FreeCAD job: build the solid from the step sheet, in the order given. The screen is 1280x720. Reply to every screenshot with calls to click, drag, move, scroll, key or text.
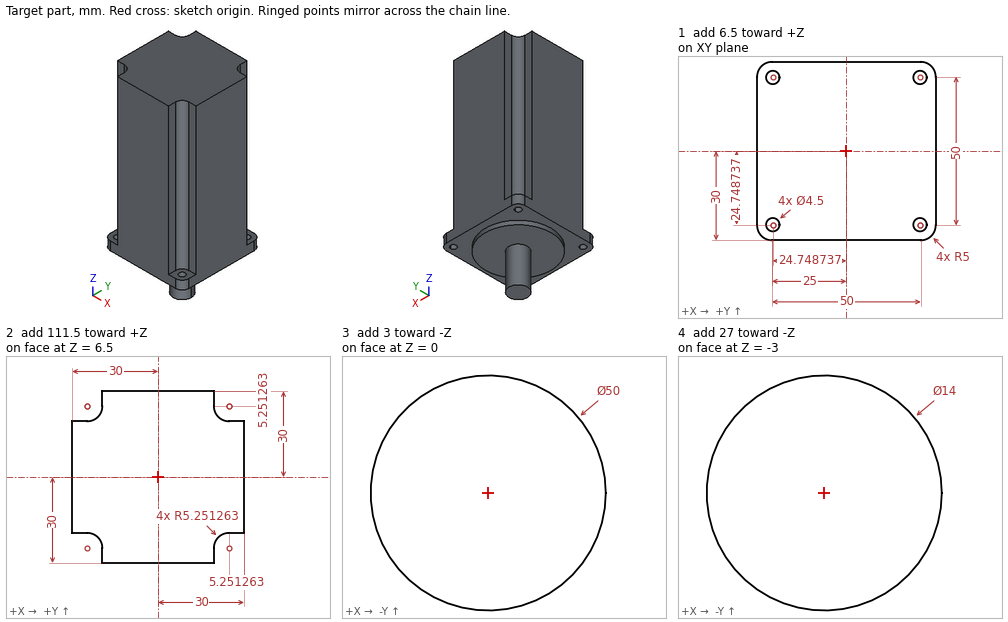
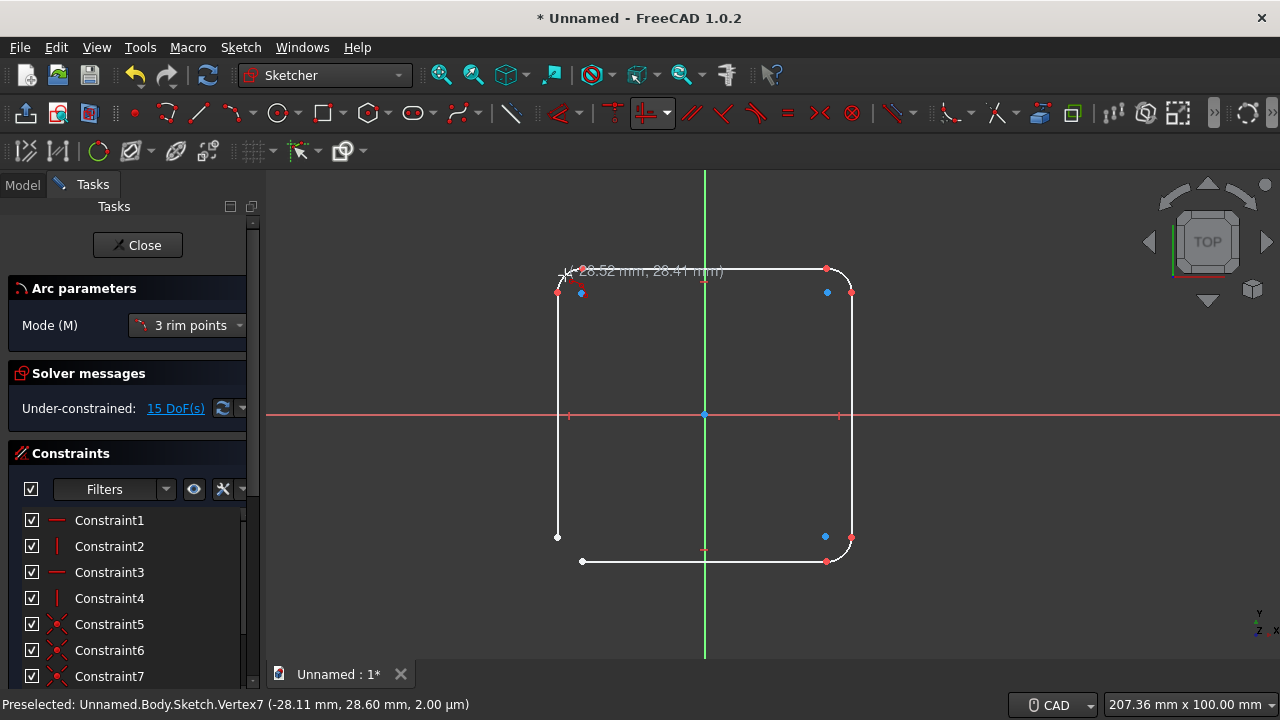
click(558, 538)
click(583, 562)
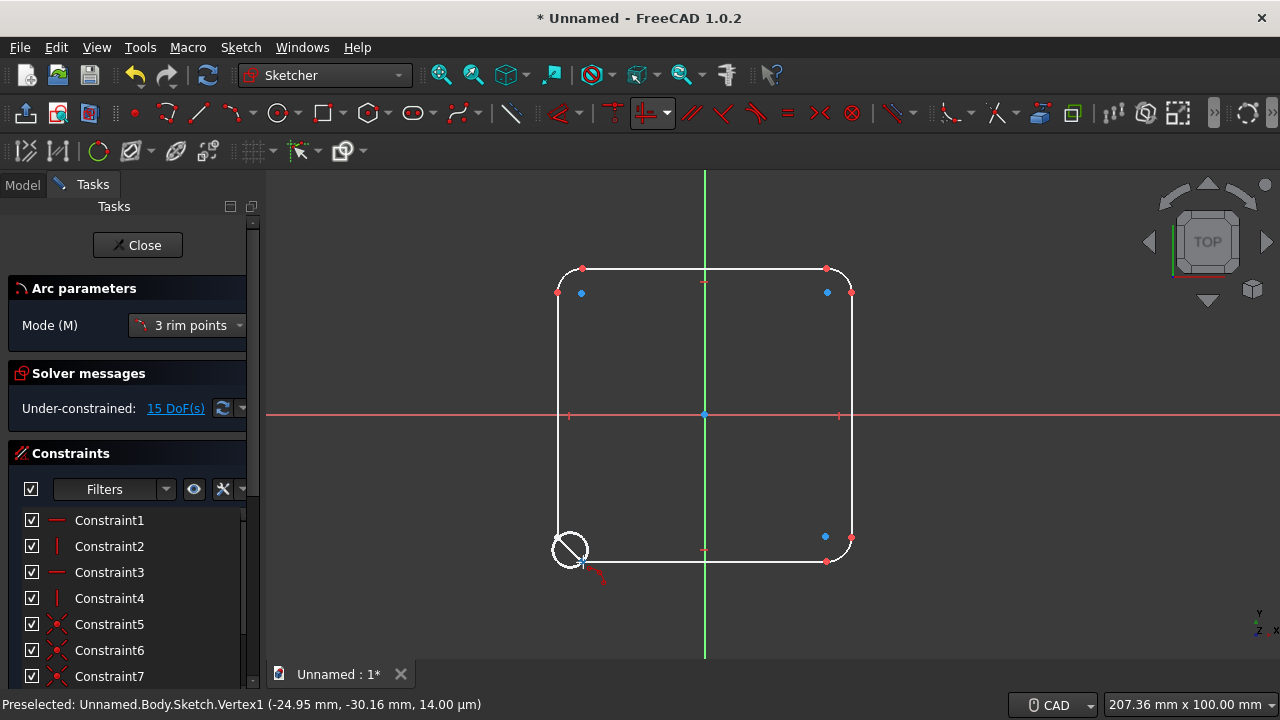
scroll(565, 554, up, 4)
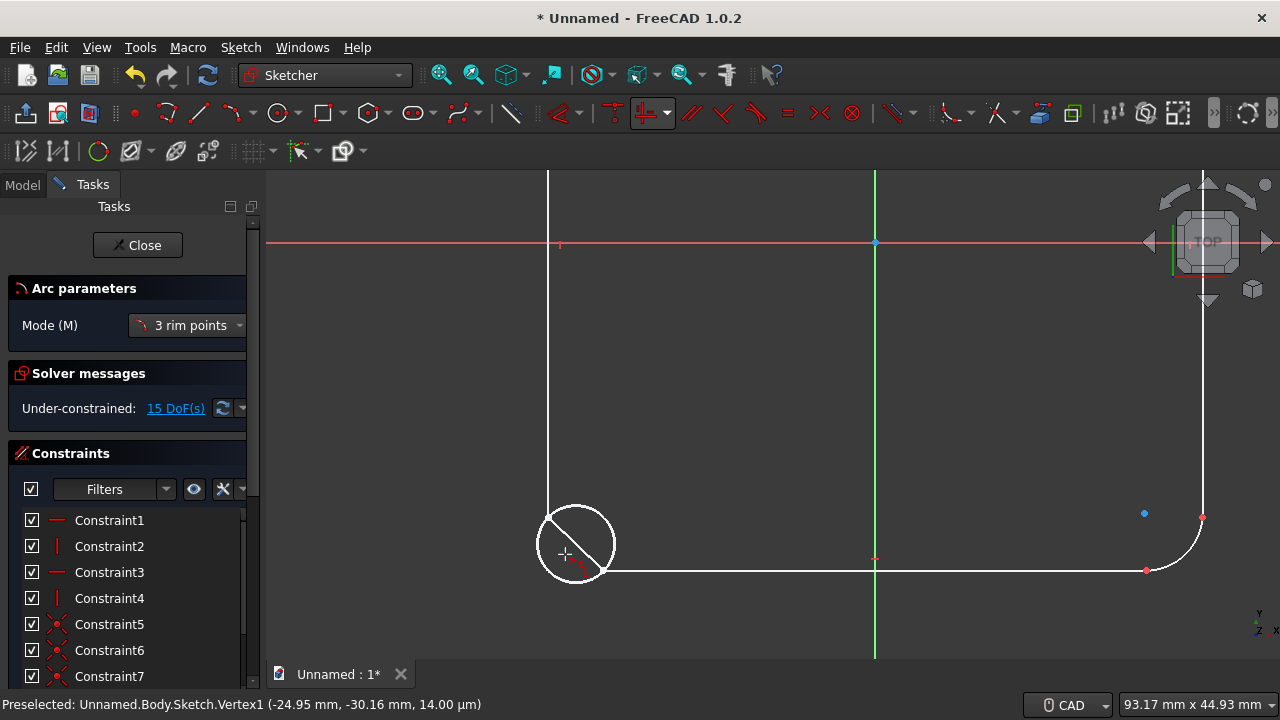
click(565, 553)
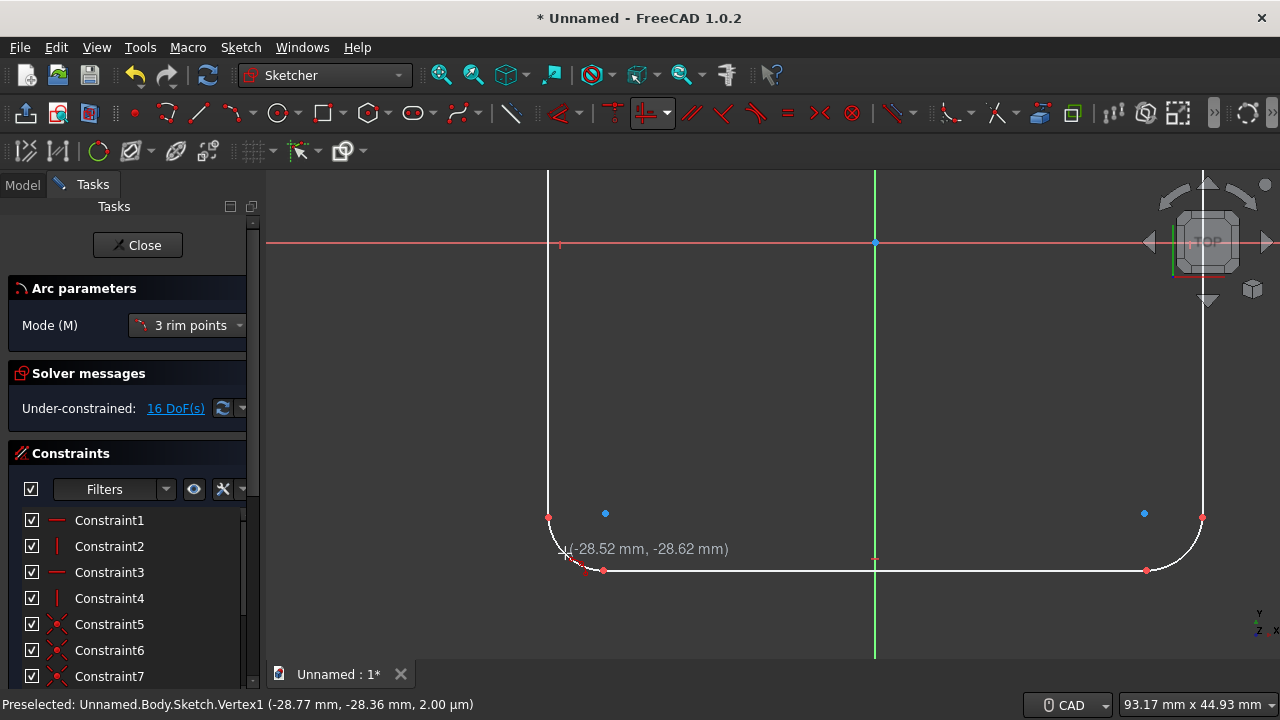
click(278, 114)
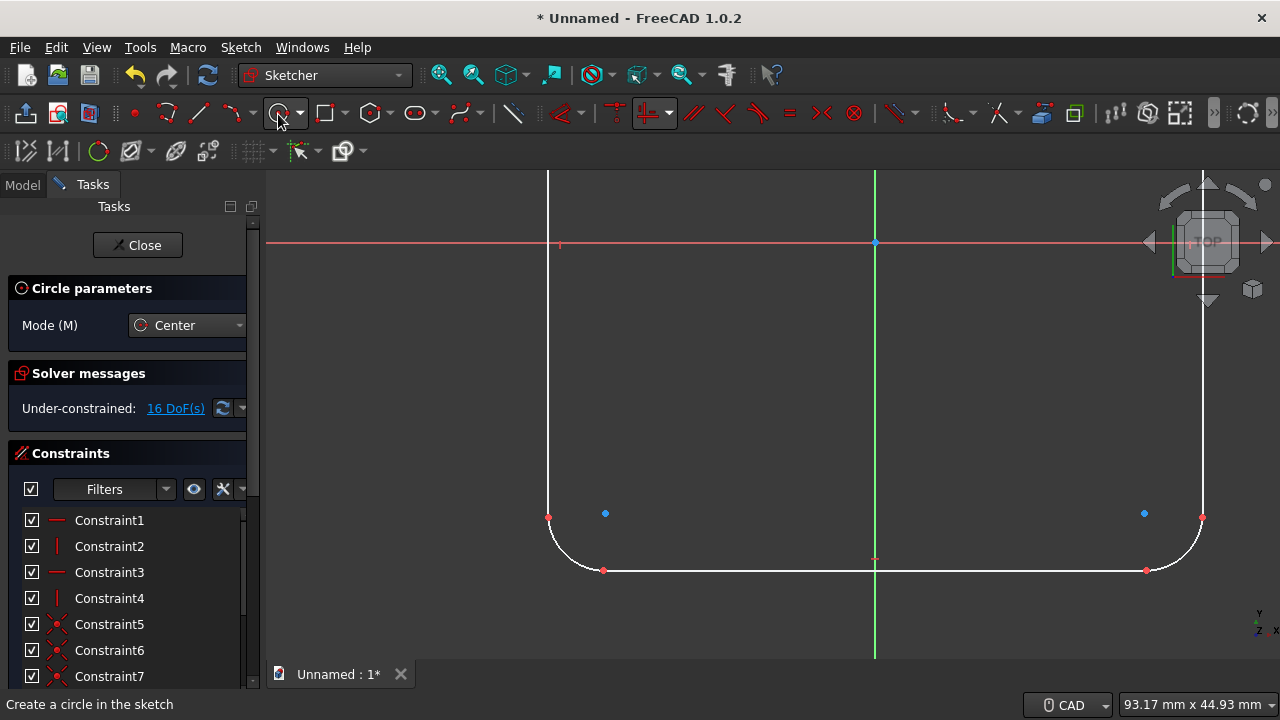
scroll(606, 512, up, 8)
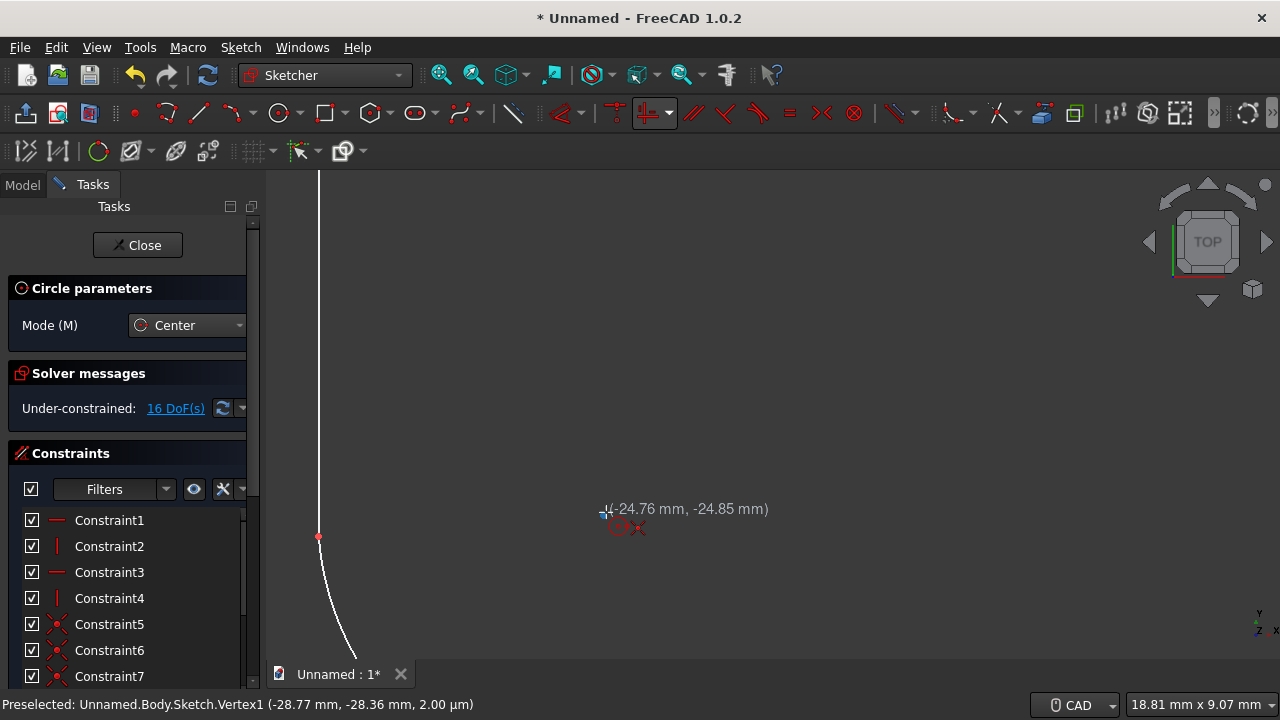
click(605, 509)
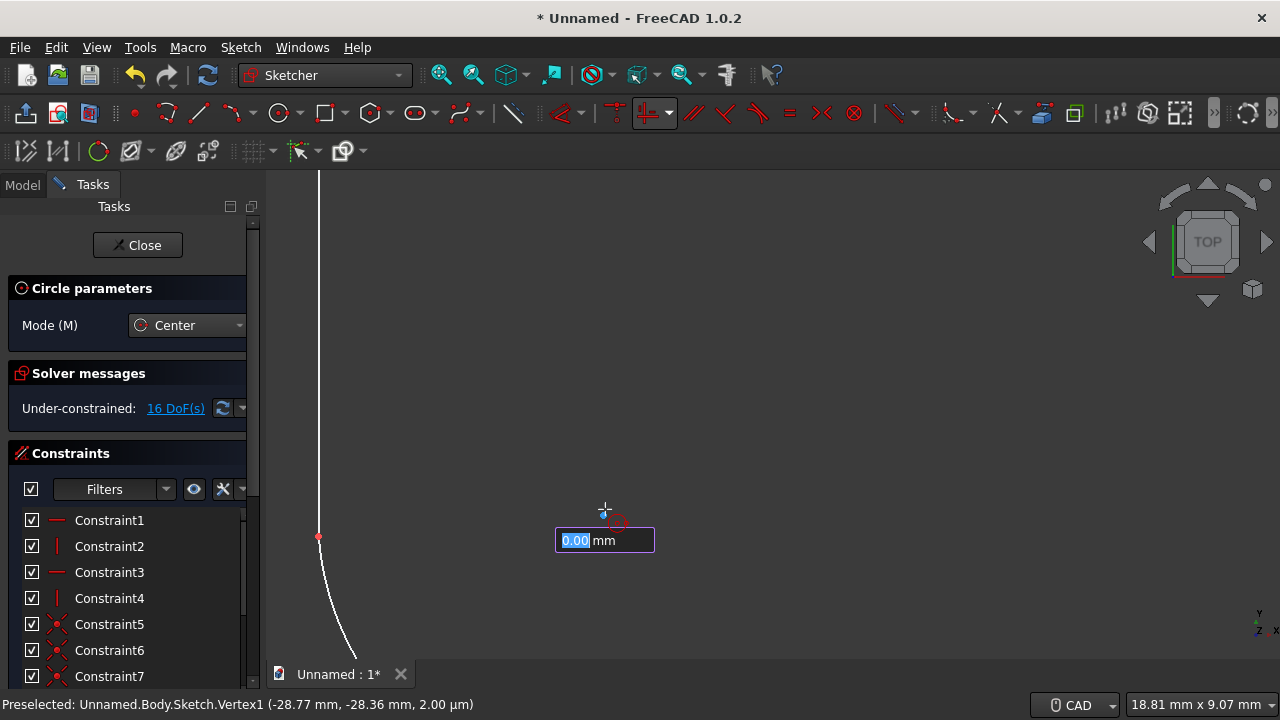
scroll(581, 538, down, 12)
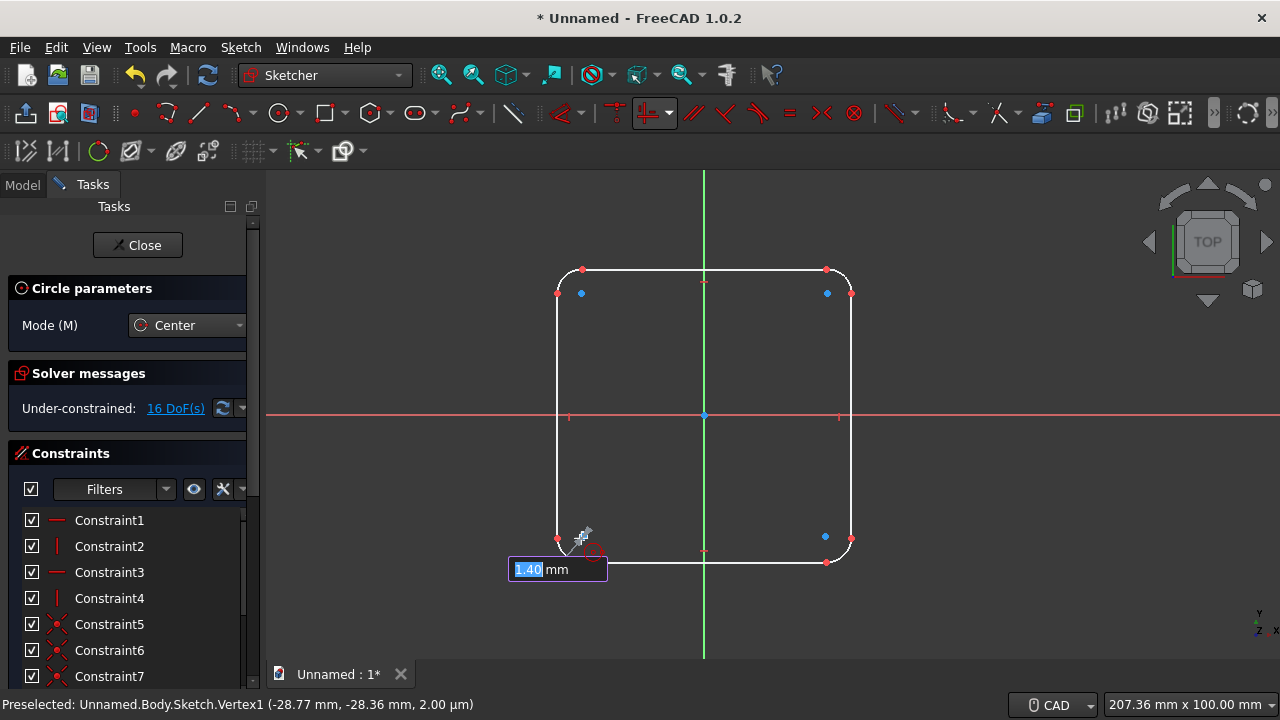
scroll(591, 528, up, 2)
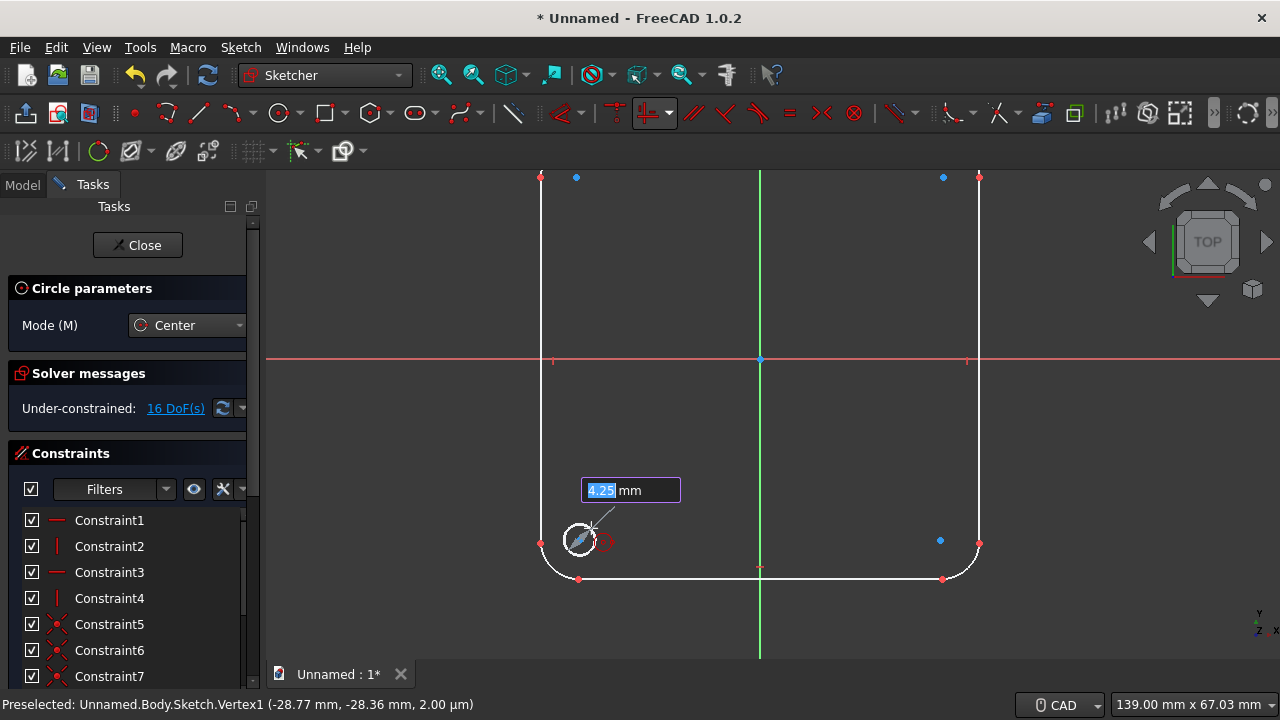
click(591, 528)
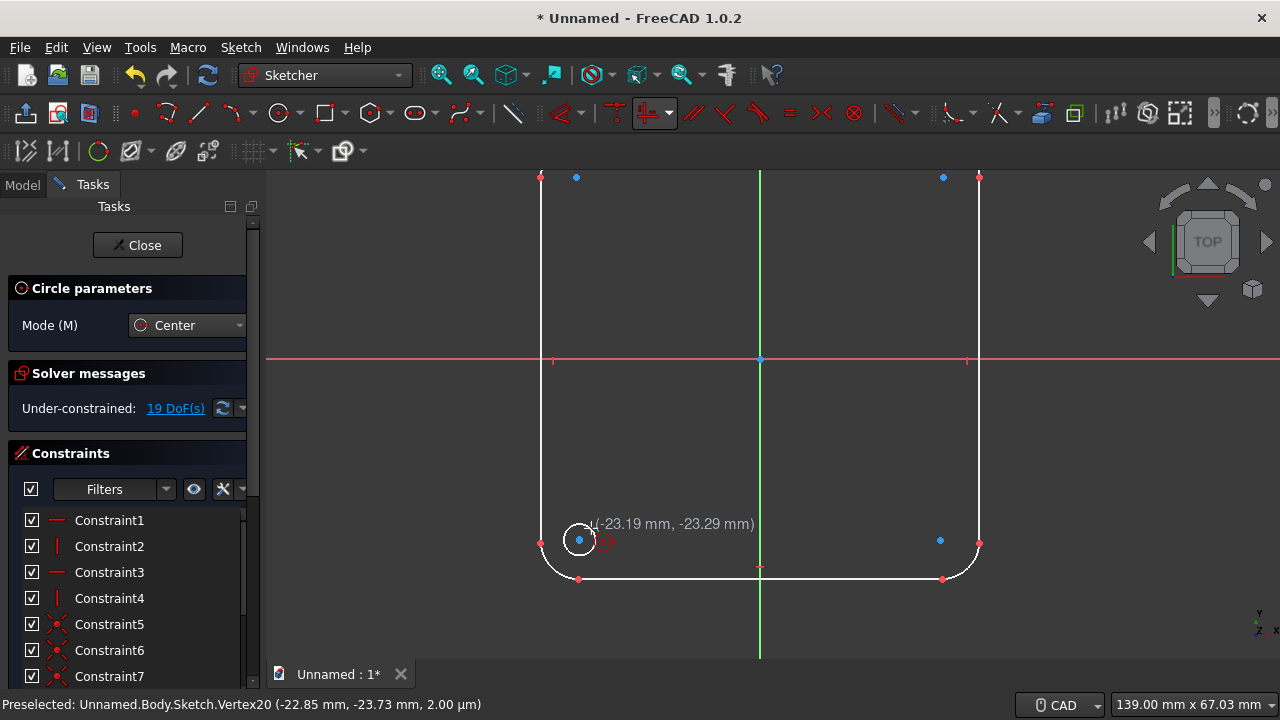
scroll(941, 540, up, 10)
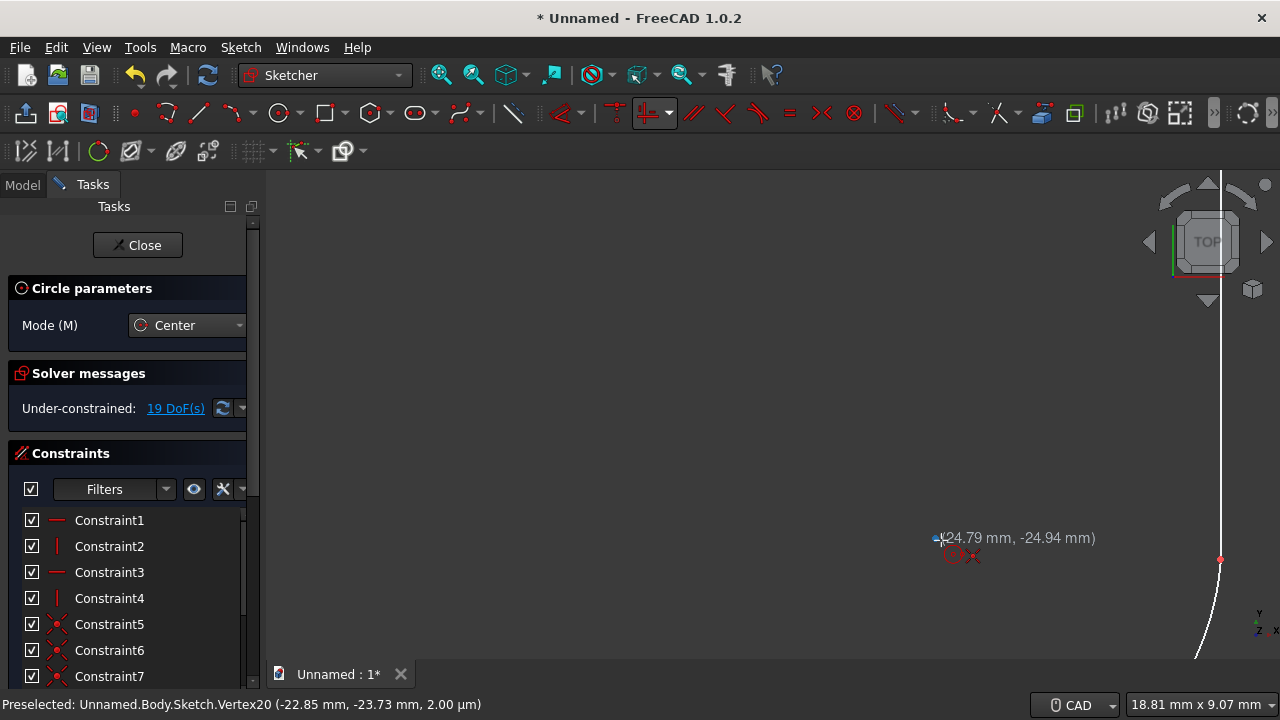
click(935, 532)